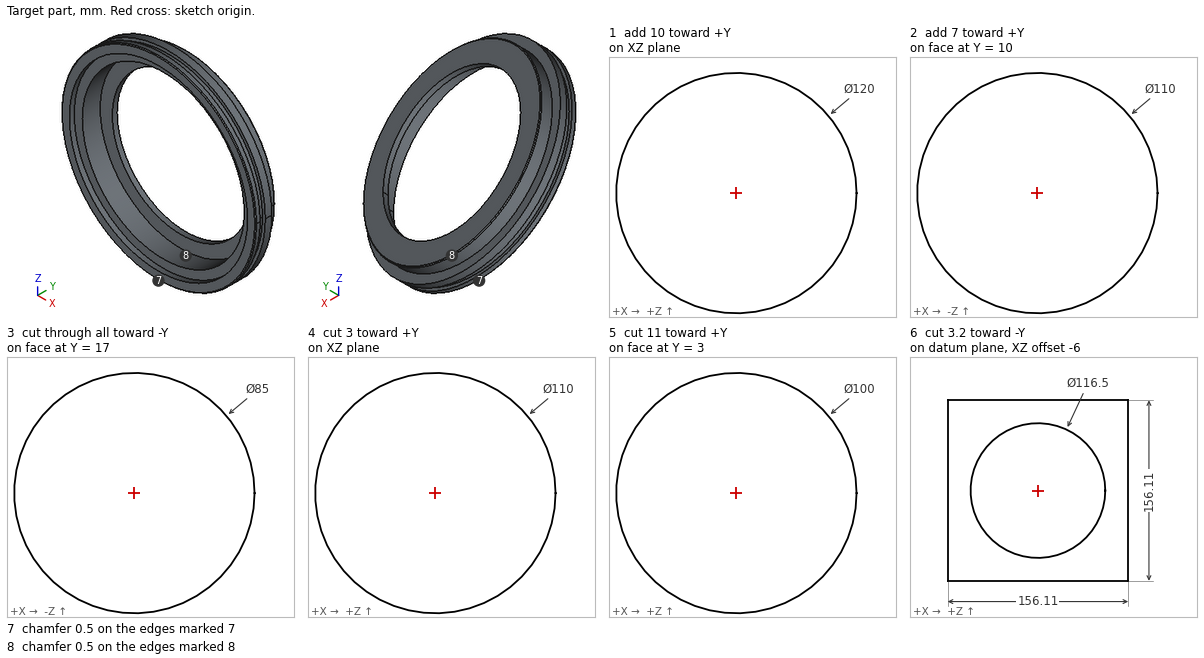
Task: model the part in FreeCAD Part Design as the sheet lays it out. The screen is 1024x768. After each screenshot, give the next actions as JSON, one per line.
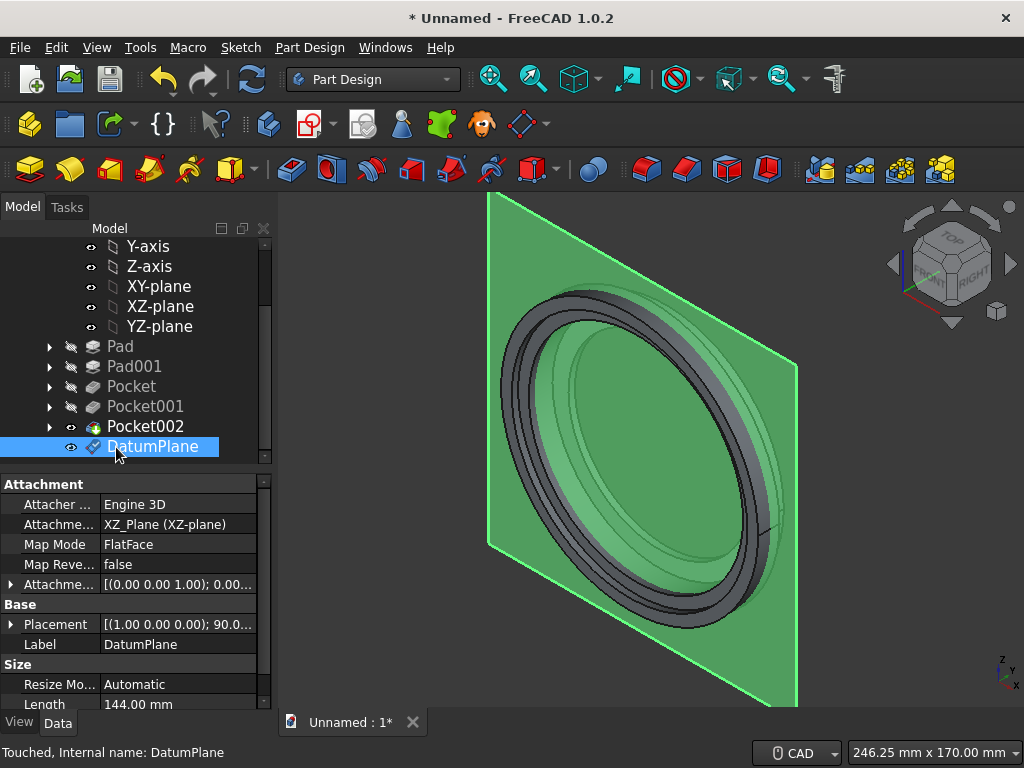
{"action": "left_click", "coordinate": [310, 124]}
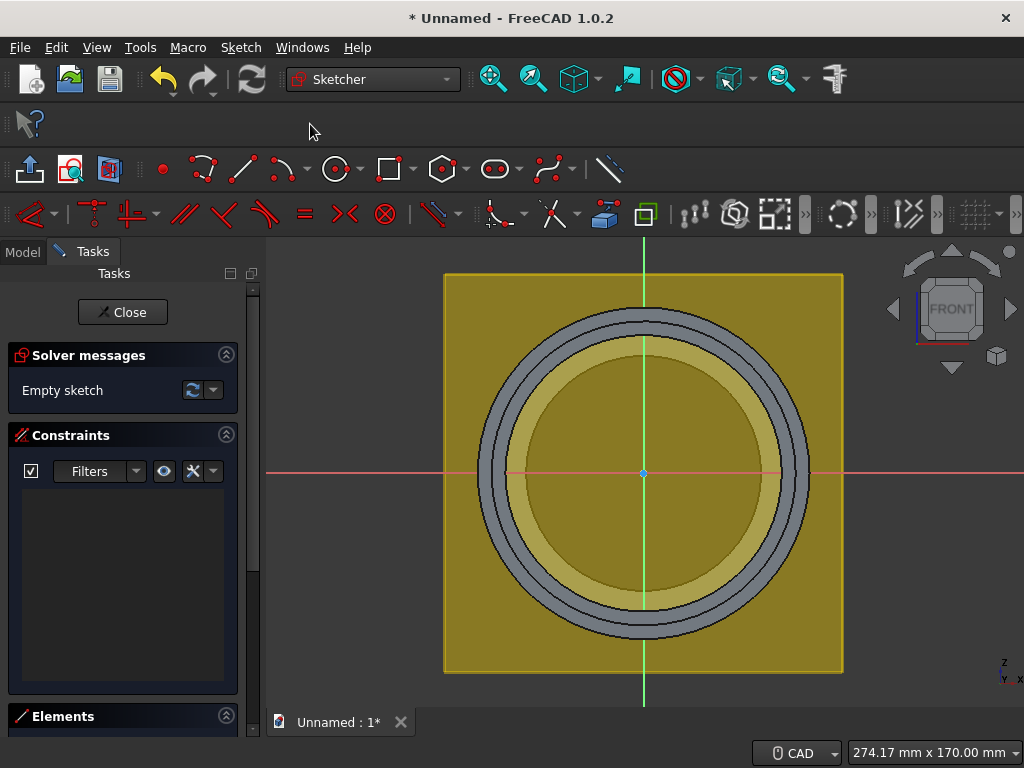
{"action": "left_click", "coordinate": [110, 170]}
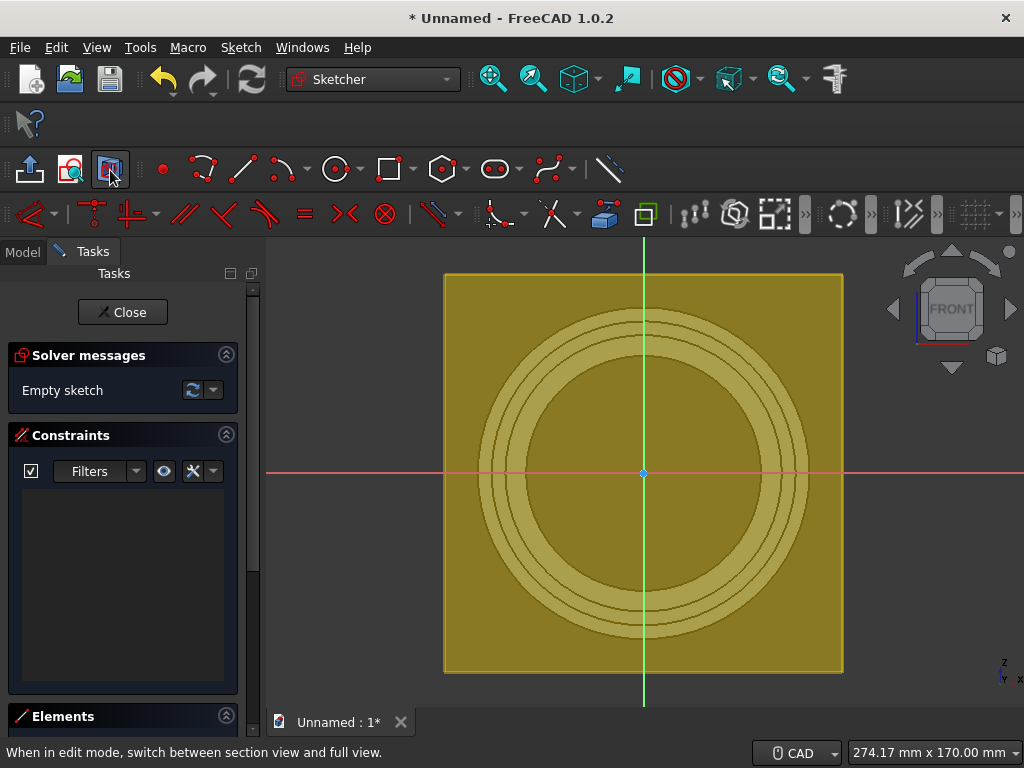
{"action": "scroll", "coordinate": [440, 469], "scroll_direction": "down", "scroll_amount": 2}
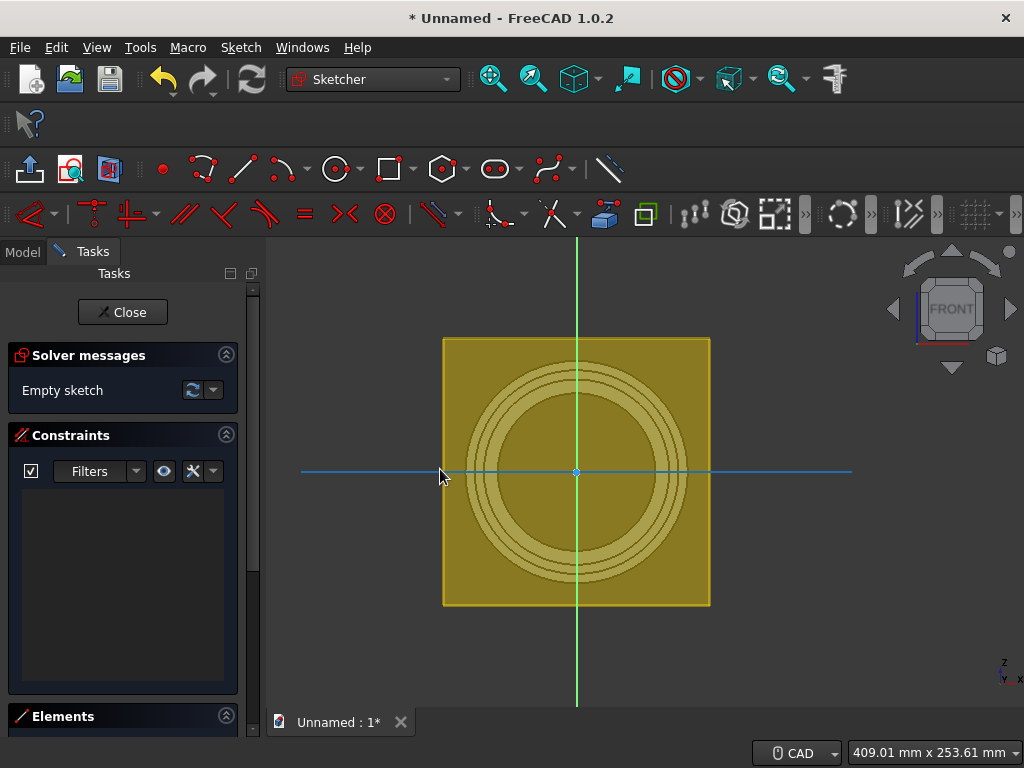
{"action": "left_click", "coordinate": [416, 170]}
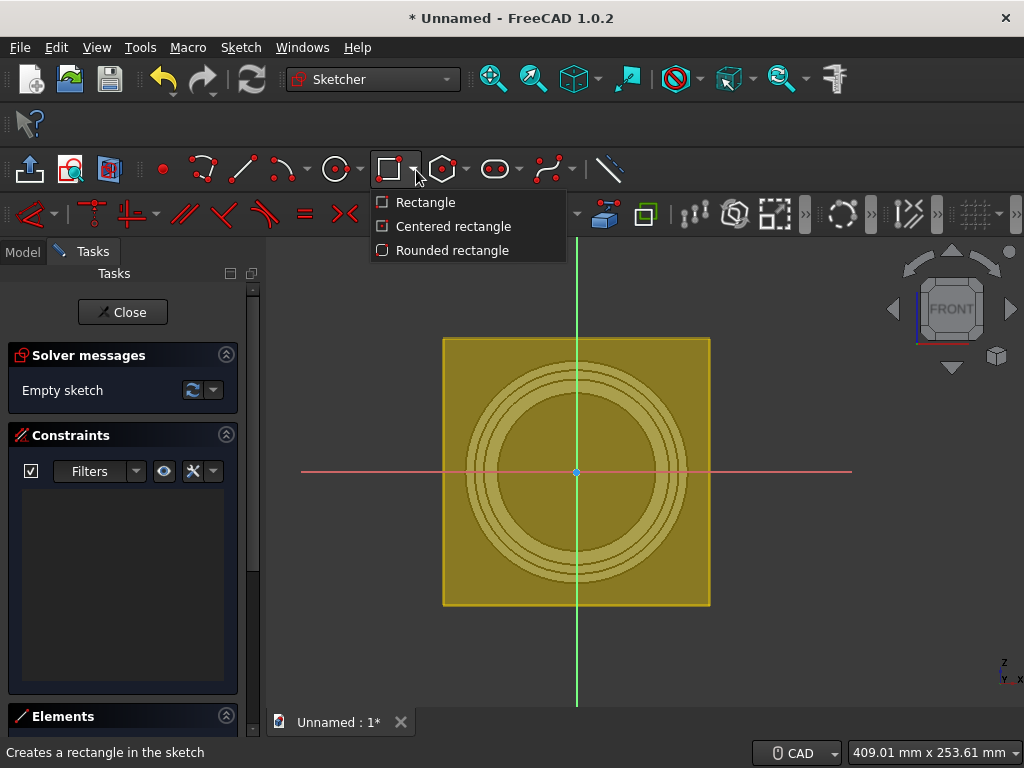
{"action": "left_click", "coordinate": [468, 226]}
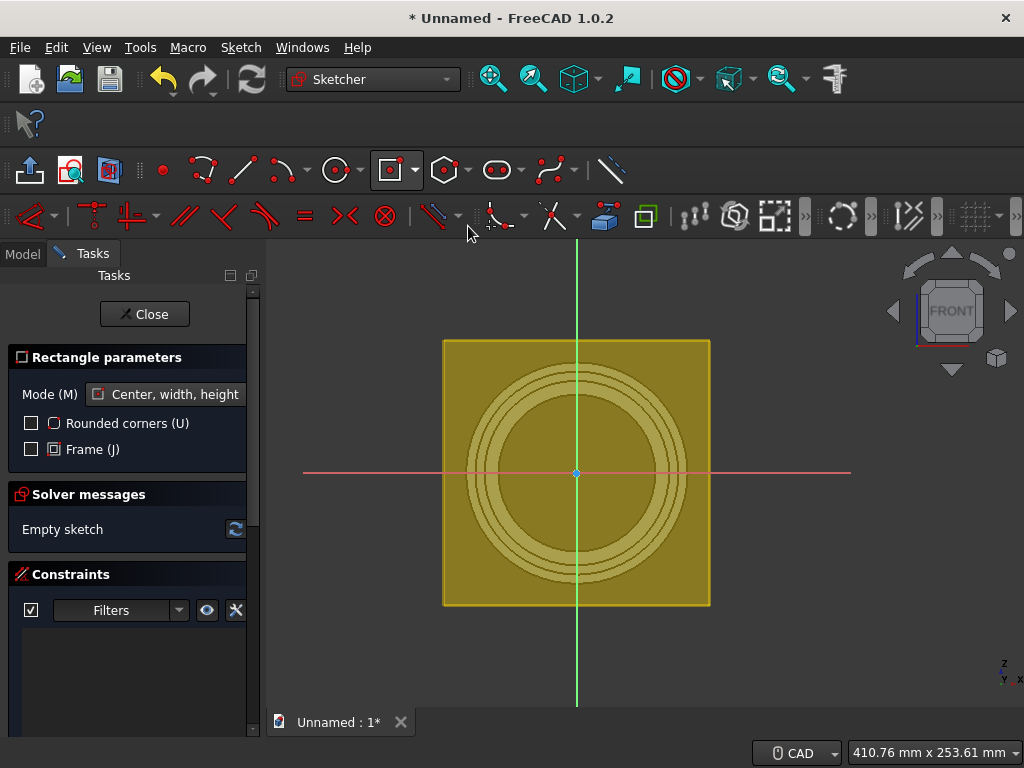
{"action": "left_click", "coordinate": [577, 473]}
{"action": "mouse_move", "coordinate": [721, 329]}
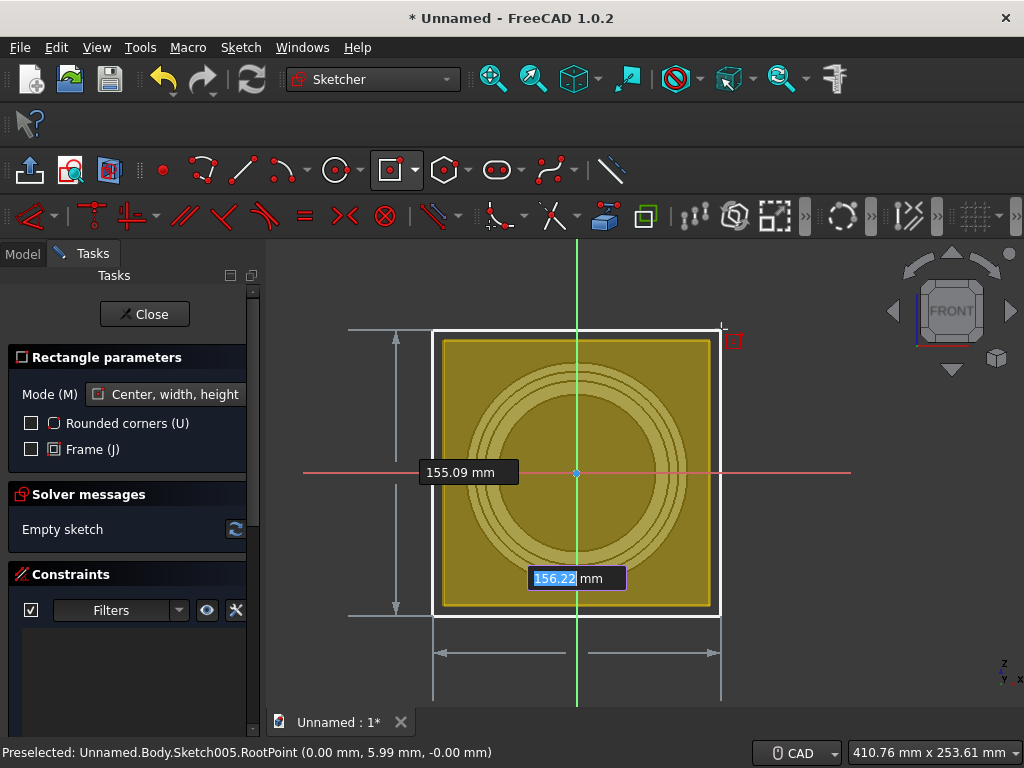
{"action": "type", "text": "156.11"}
{"action": "key", "text": "Tab"}
{"action": "type", "text": "156.11"}
{"action": "key", "text": "Return"}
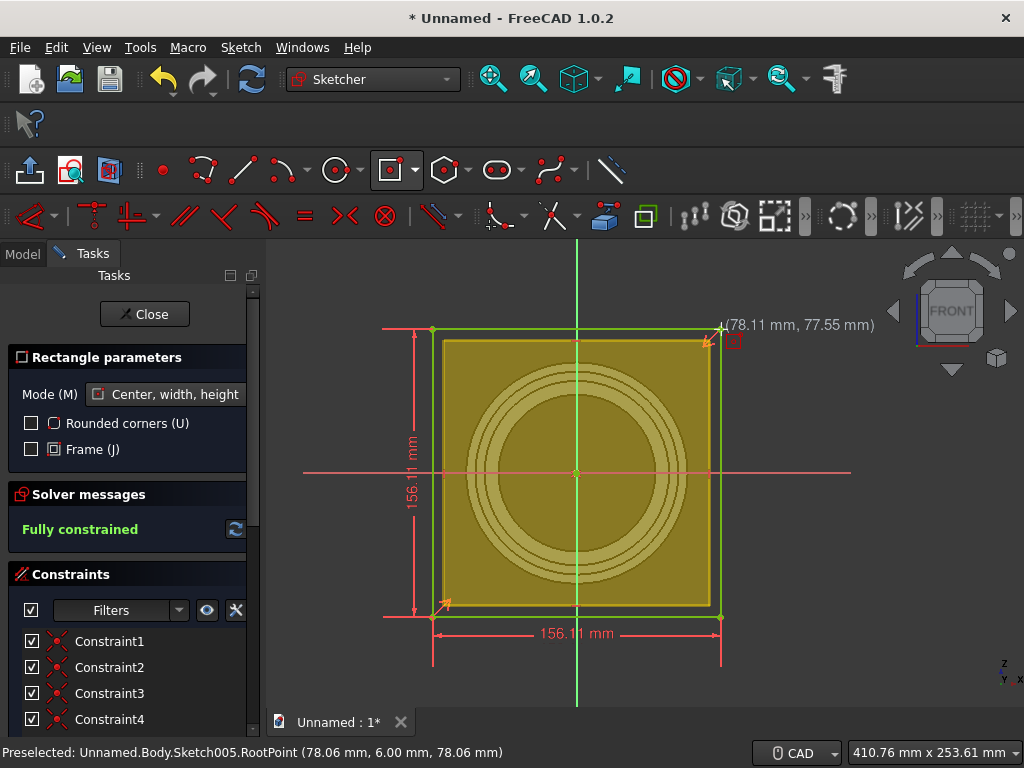
{"action": "left_click", "coordinate": [336, 170]}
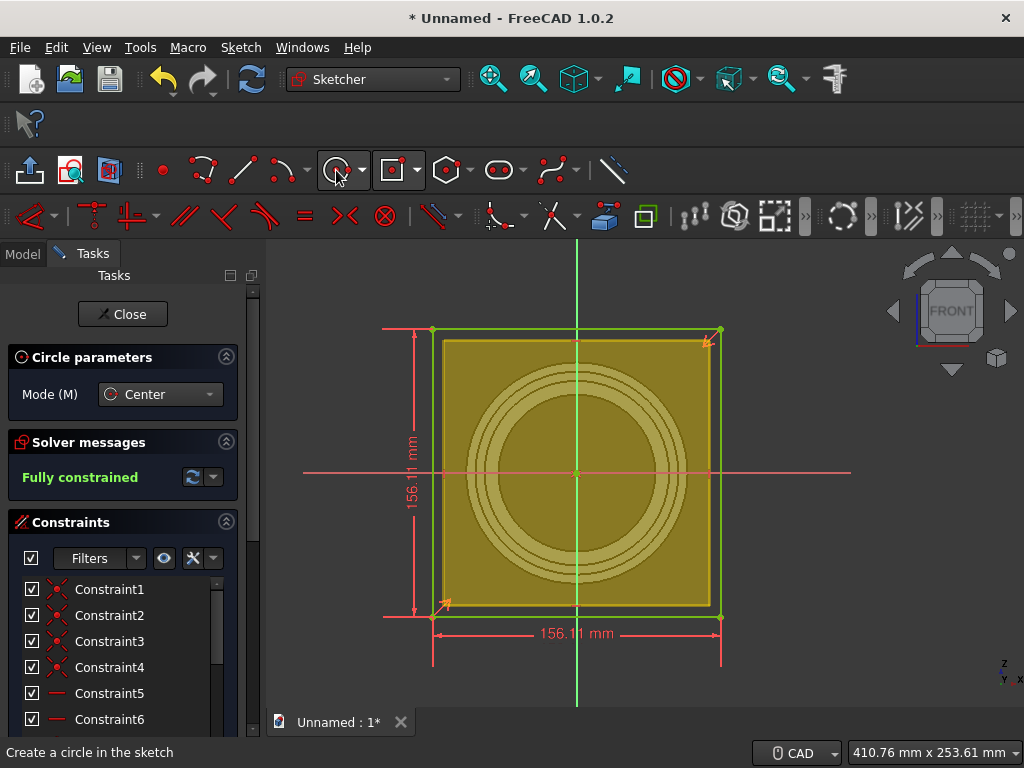
{"action": "left_click", "coordinate": [577, 473]}
{"action": "mouse_move", "coordinate": [653, 397]}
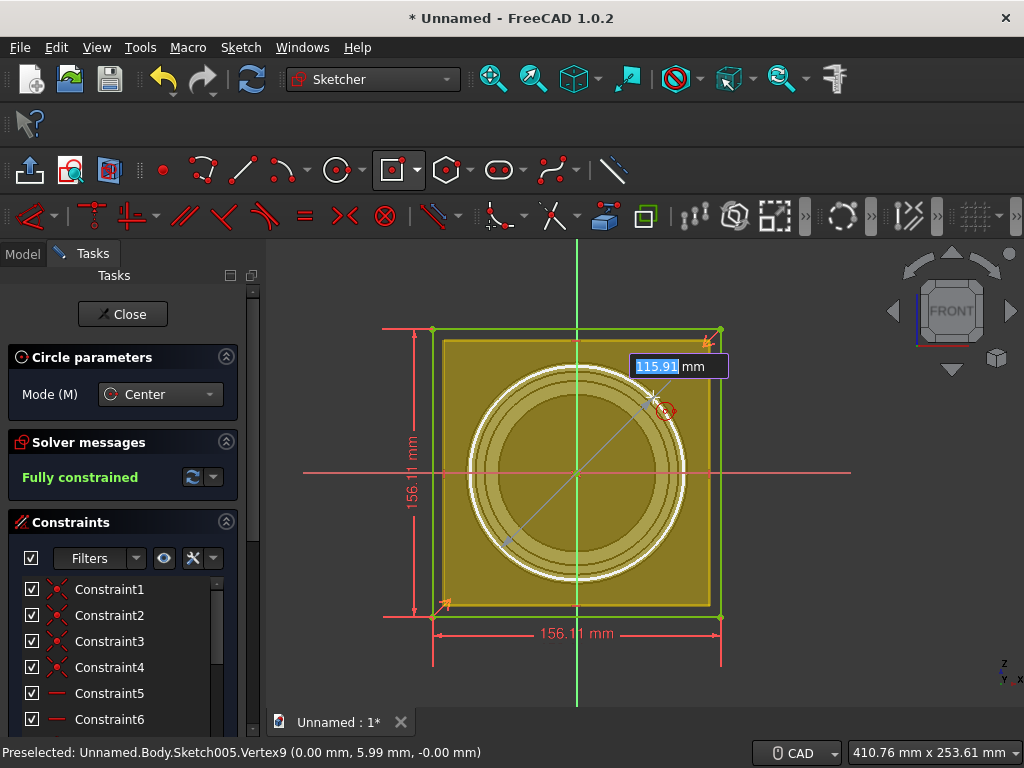
{"action": "type", "text": "116.5"}
{"action": "key", "text": "Return"}
{"action": "key", "text": "Escape"}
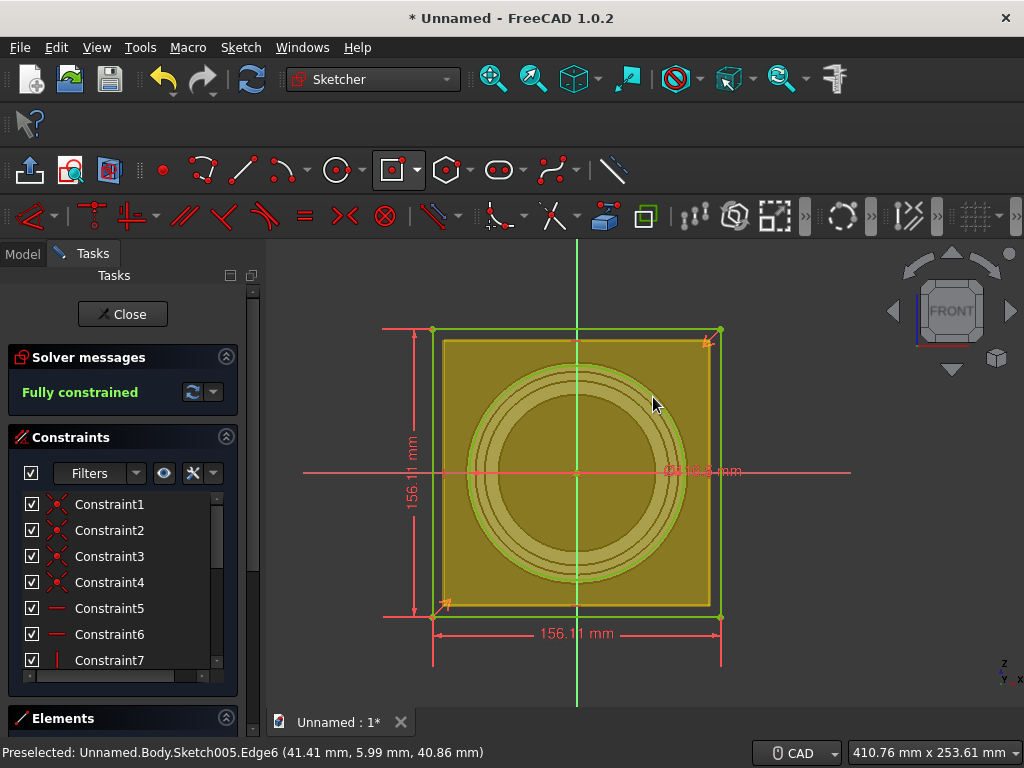
{"action": "left_click", "coordinate": [123, 314]}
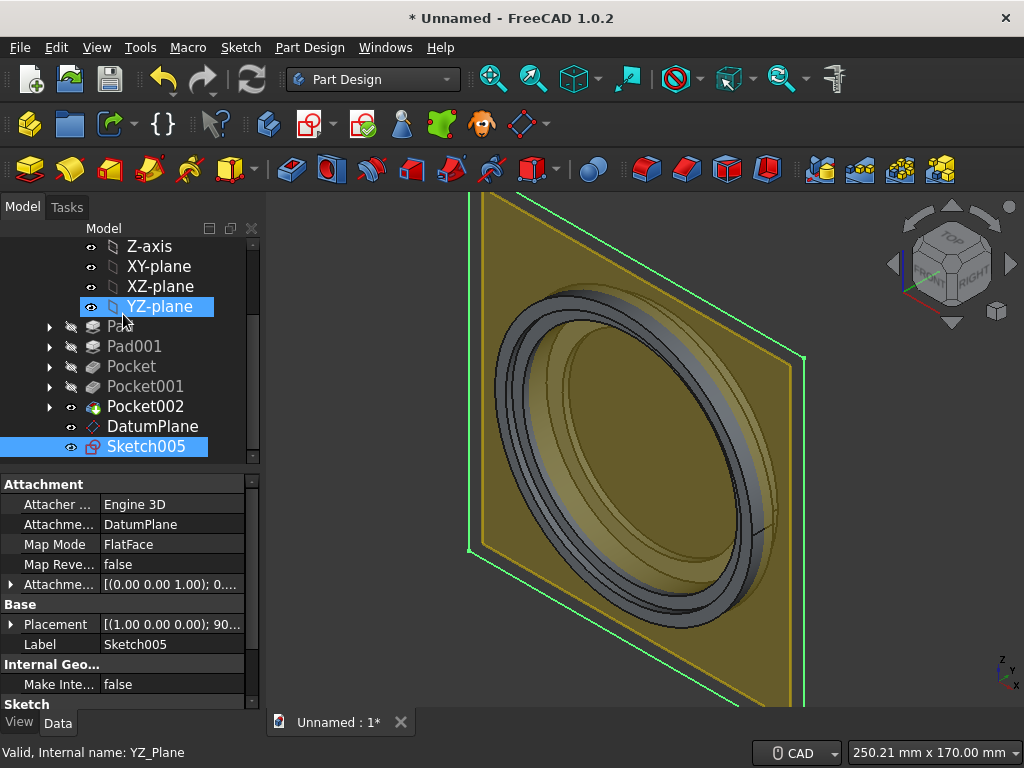
{"action": "left_click", "coordinate": [292, 170]}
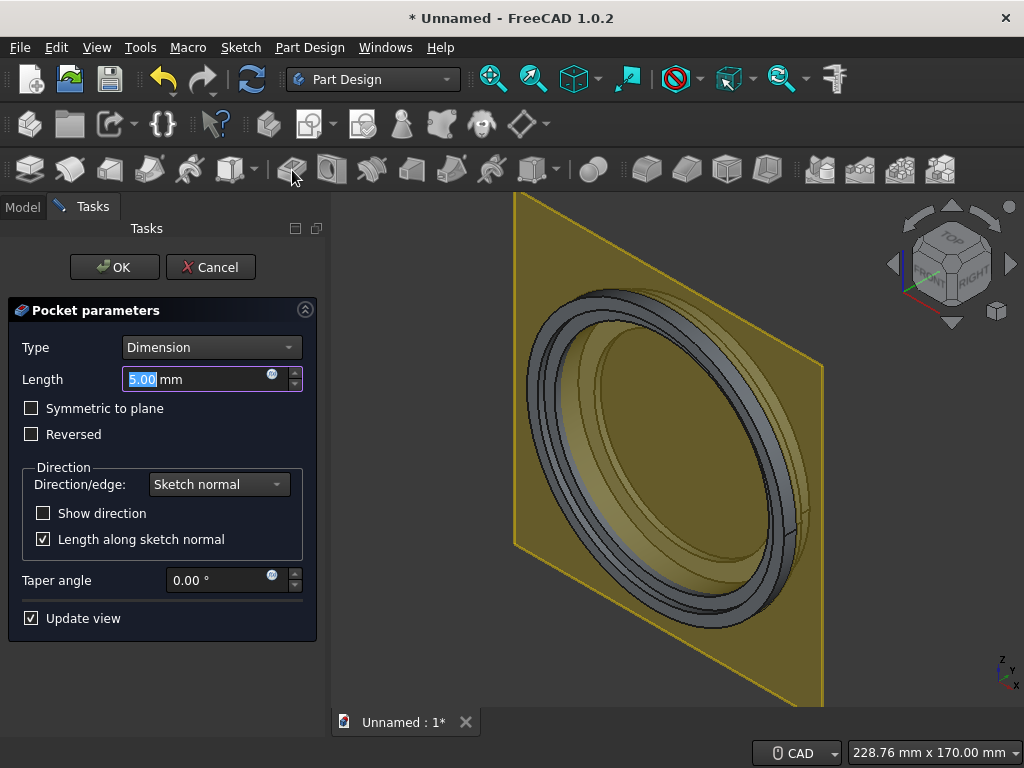
{"action": "type", "text": "3.2"}
{"action": "key", "text": "Tab"}